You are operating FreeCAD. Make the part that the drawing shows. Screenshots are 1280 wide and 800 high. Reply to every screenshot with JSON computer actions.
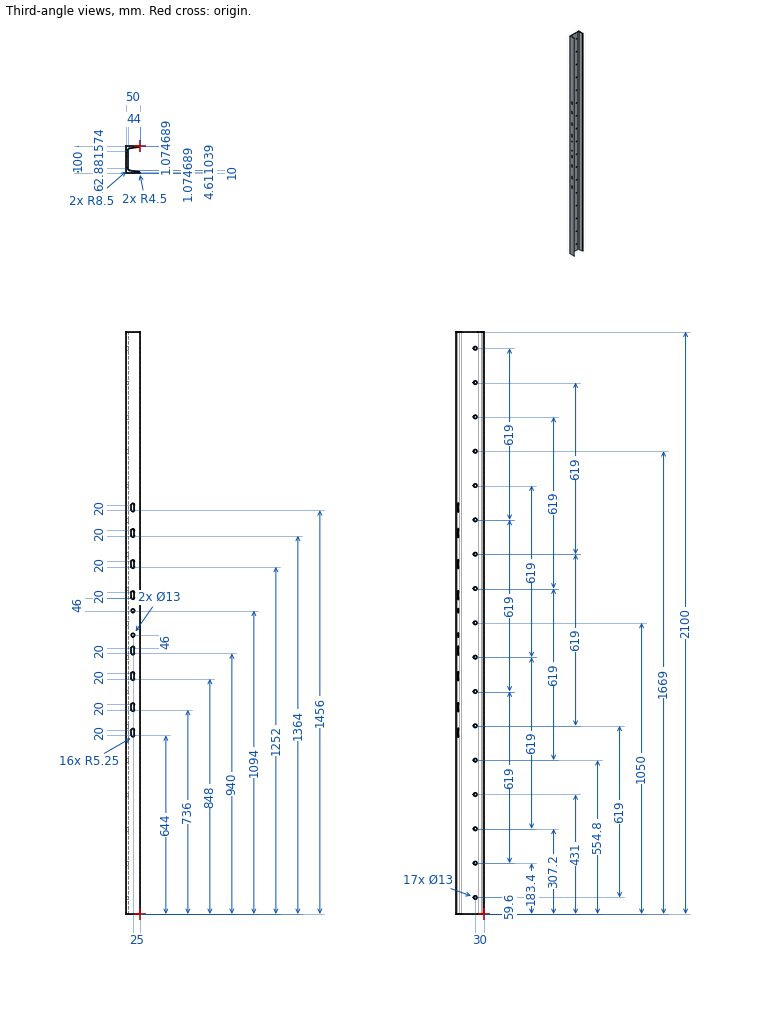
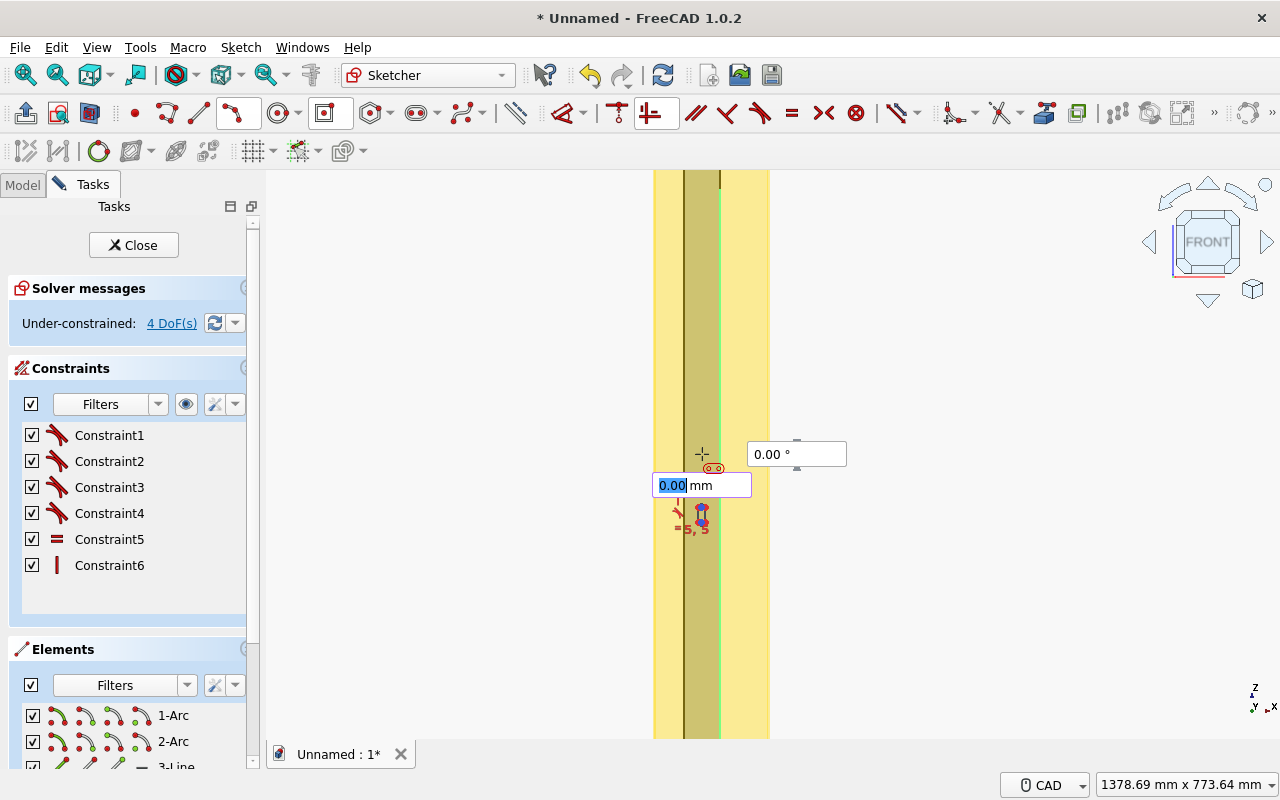
{"action": "left_click", "coordinate": [702, 439]}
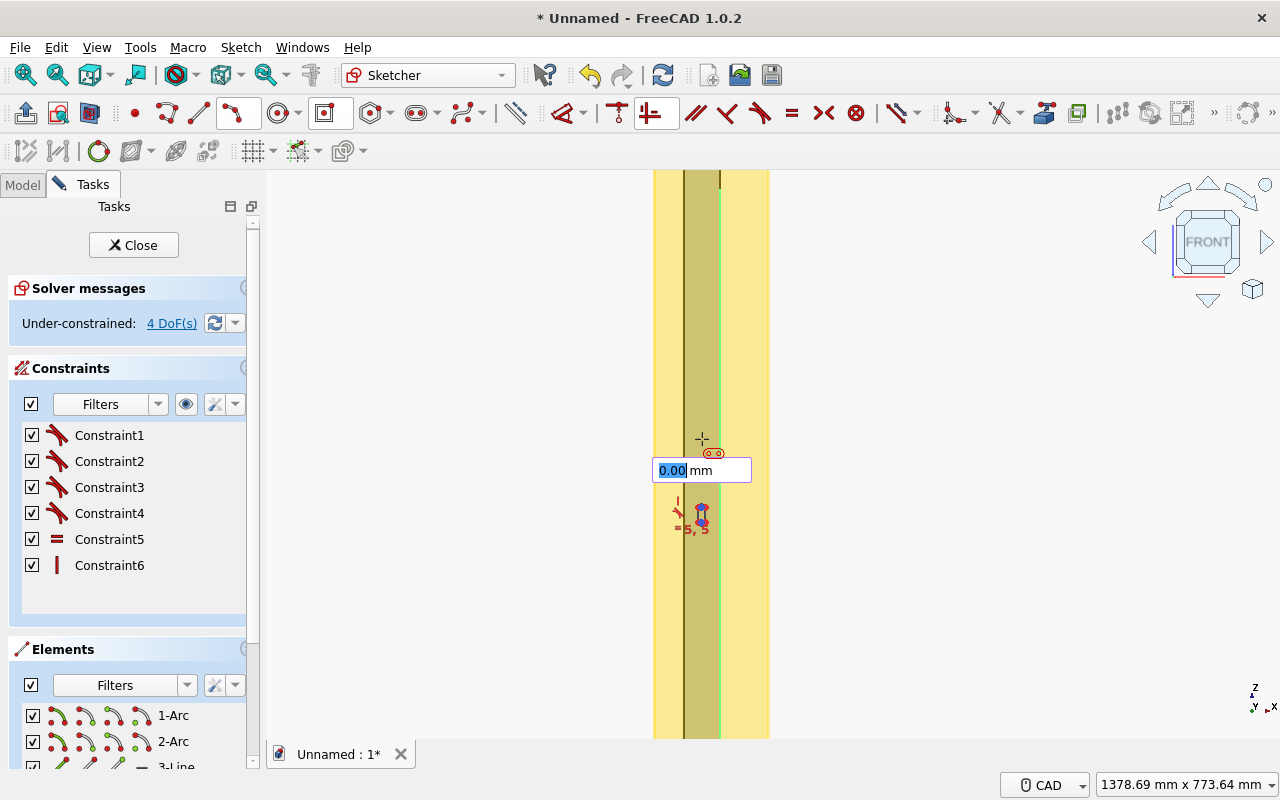
{"action": "scroll", "coordinate": [698, 447], "scroll_direction": "up", "scroll_amount": 8}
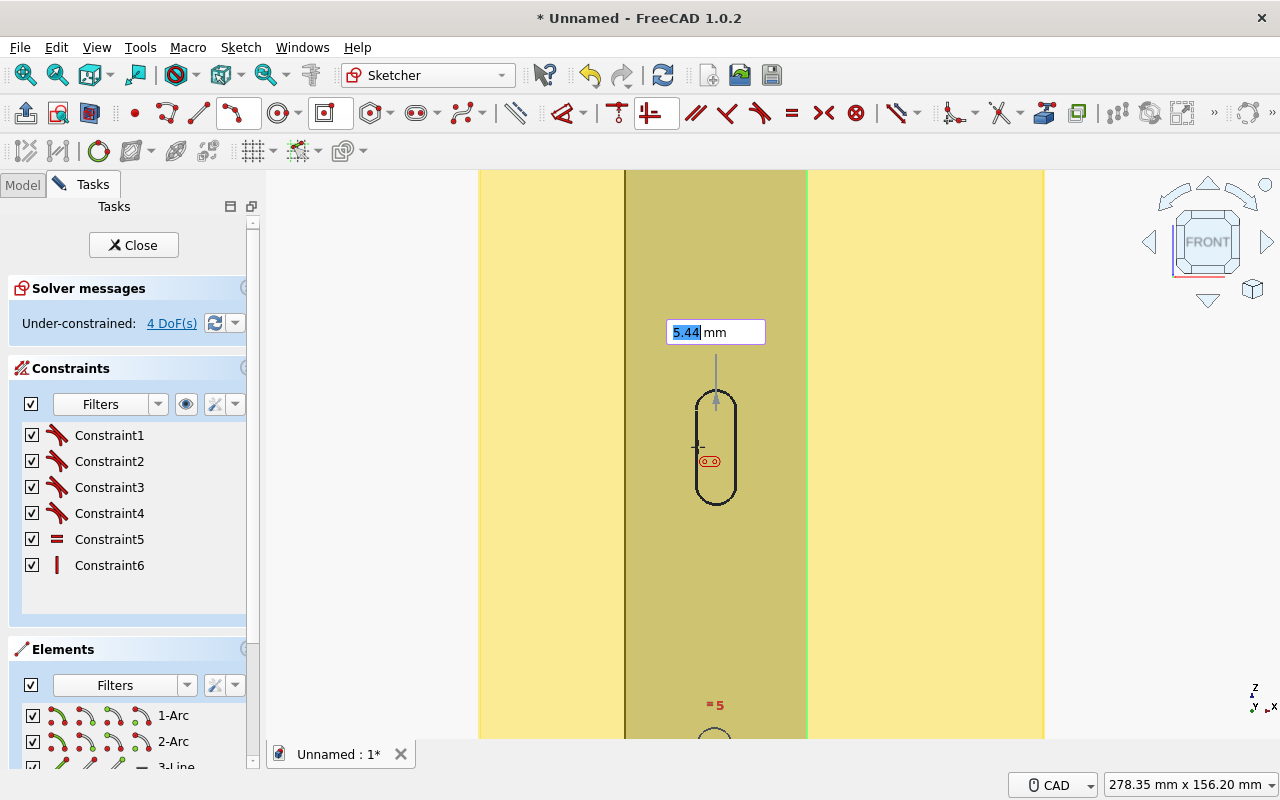
{"action": "left_click", "coordinate": [697, 443]}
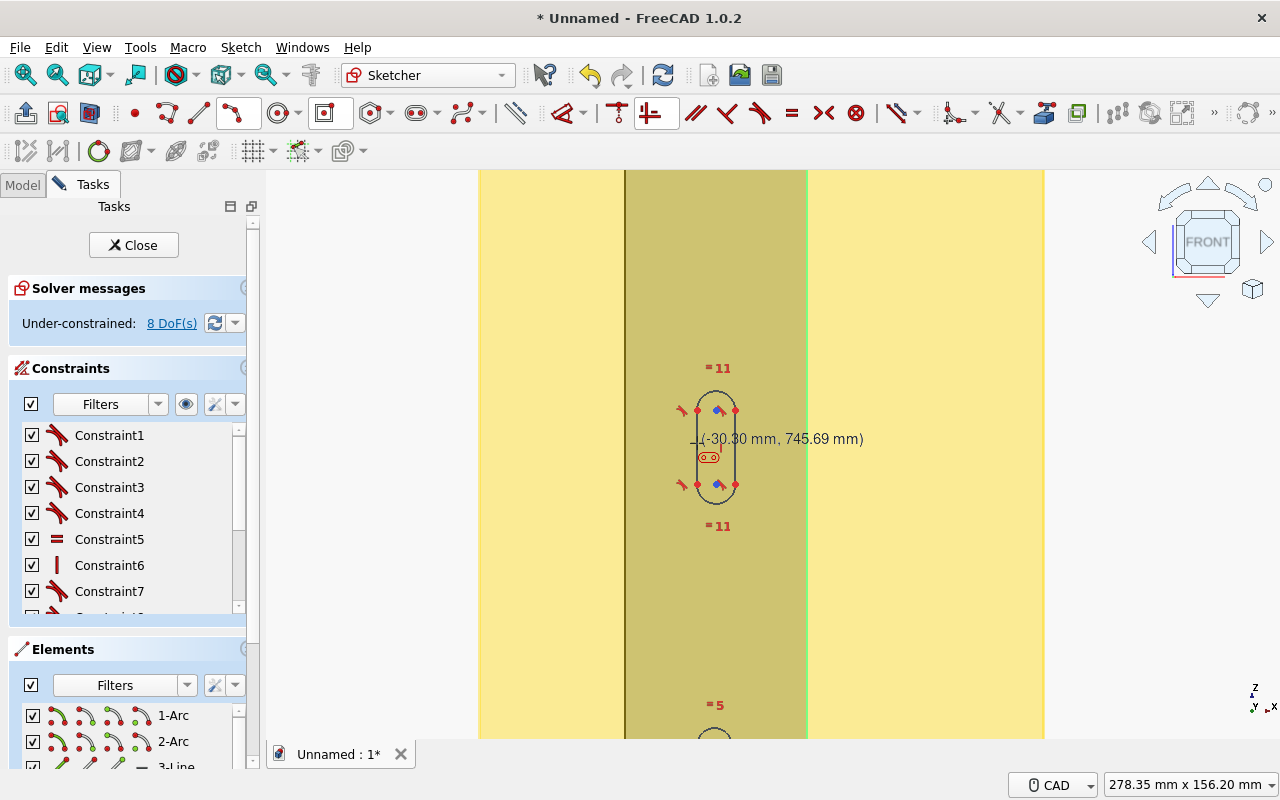
{"action": "scroll", "coordinate": [702, 454], "scroll_direction": "down", "scroll_amount": 14}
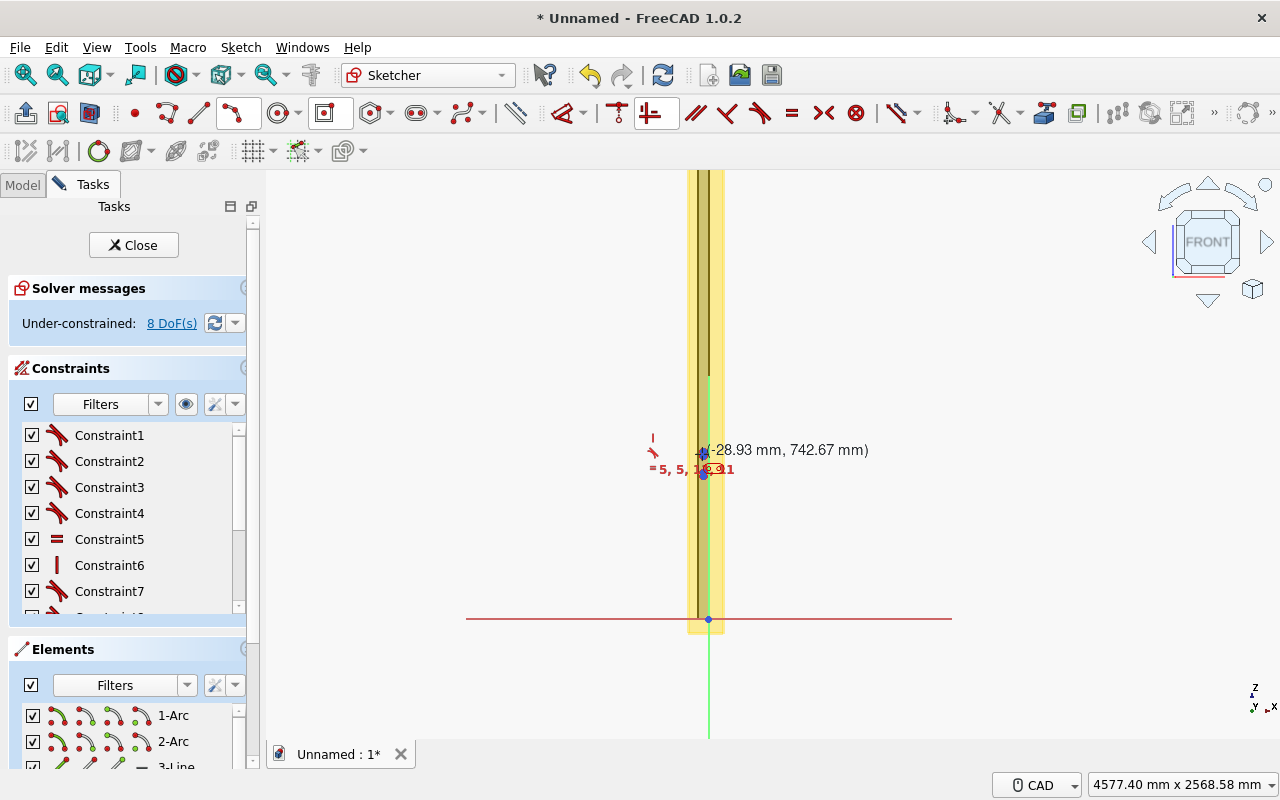
{"action": "scroll", "coordinate": [703, 431], "scroll_direction": "up", "scroll_amount": 15}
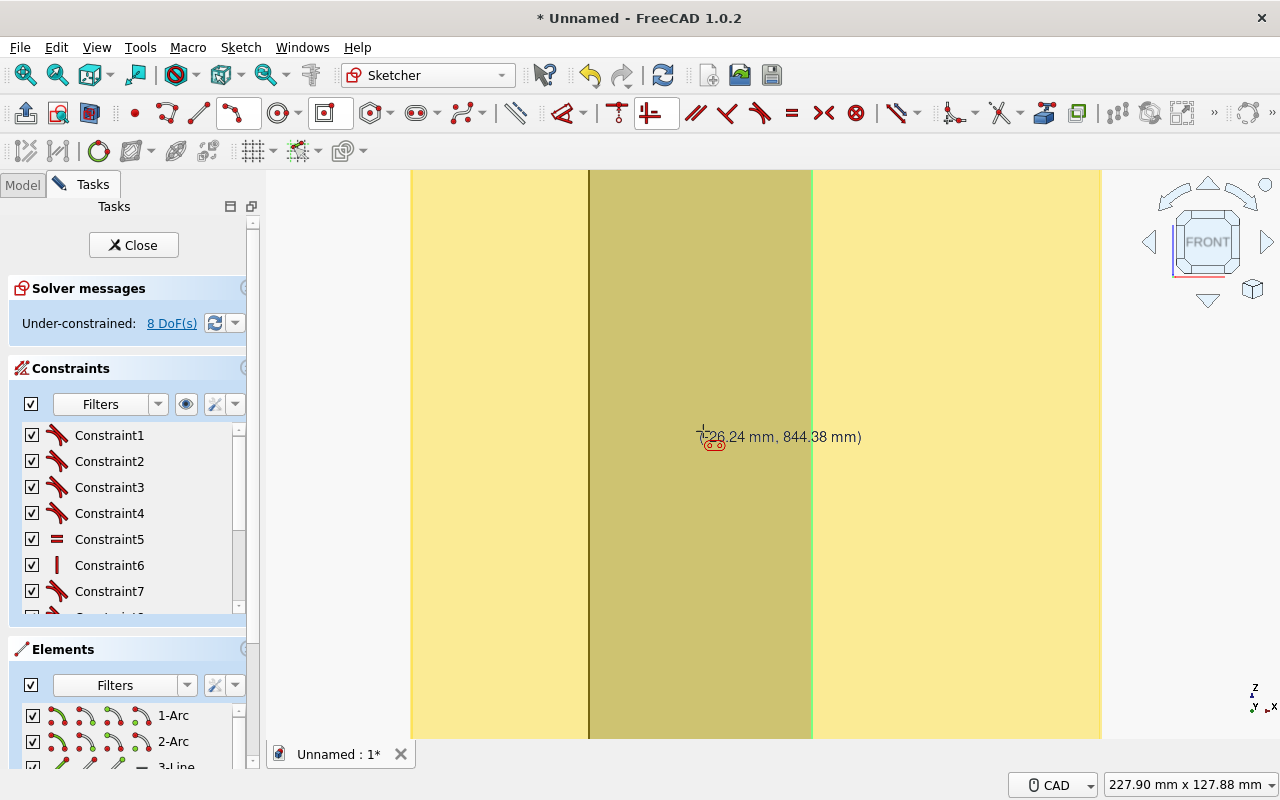
{"action": "scroll", "coordinate": [703, 431], "scroll_direction": "down", "scroll_amount": 15}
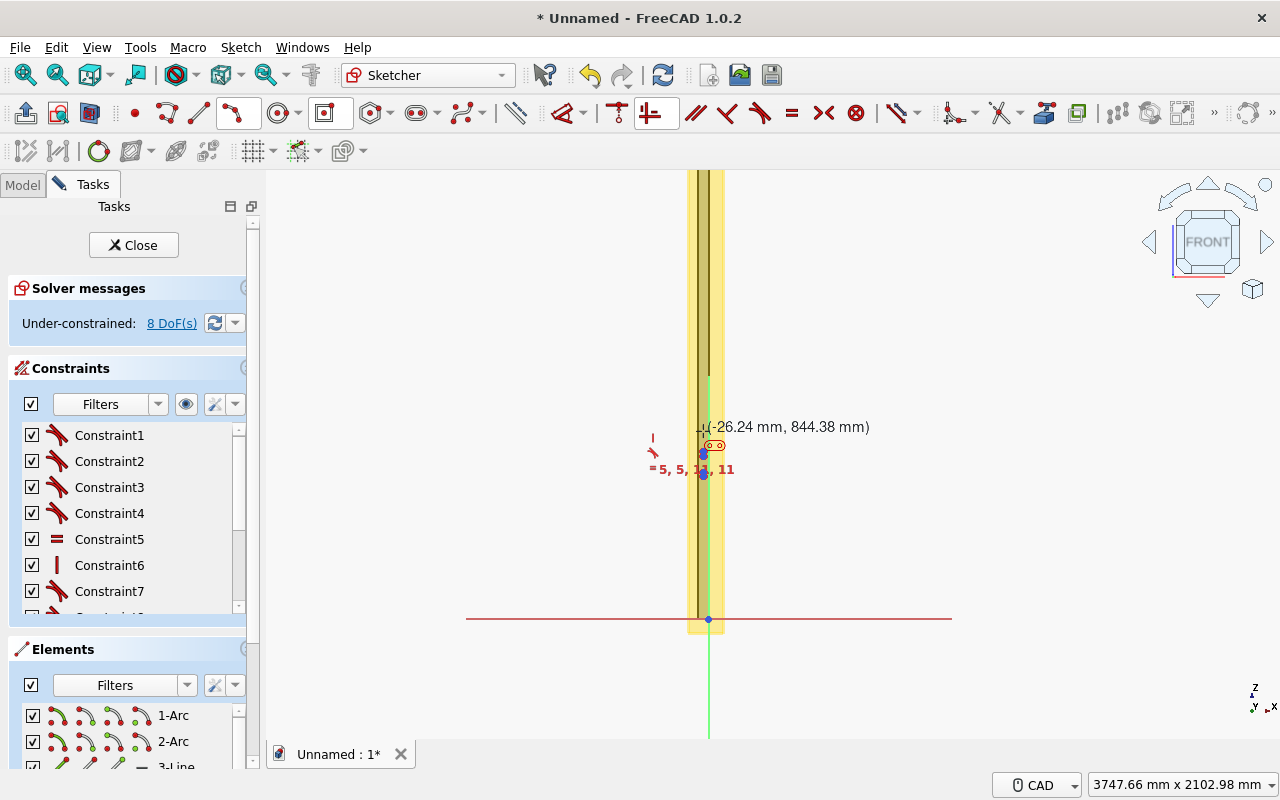
{"action": "scroll", "coordinate": [703, 431], "scroll_direction": "up", "scroll_amount": 6}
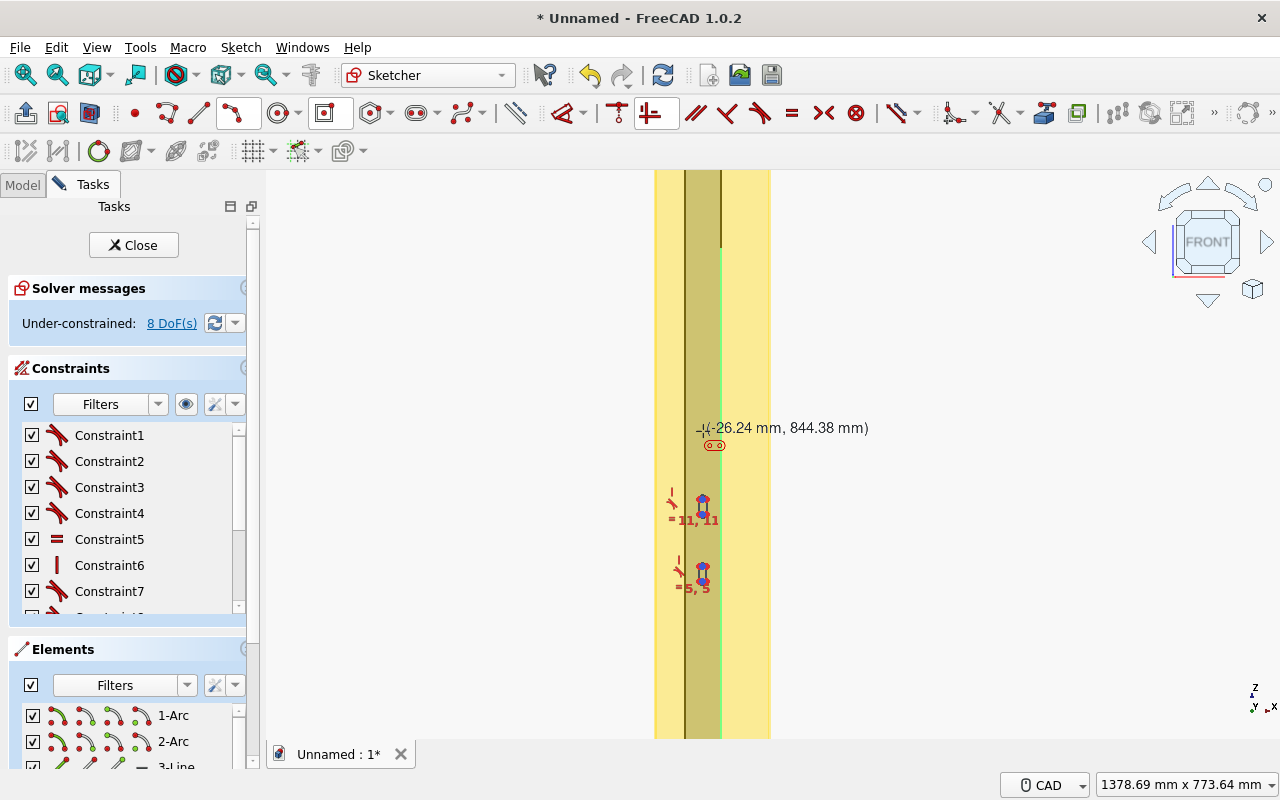
{"action": "left_click", "coordinate": [703, 431]}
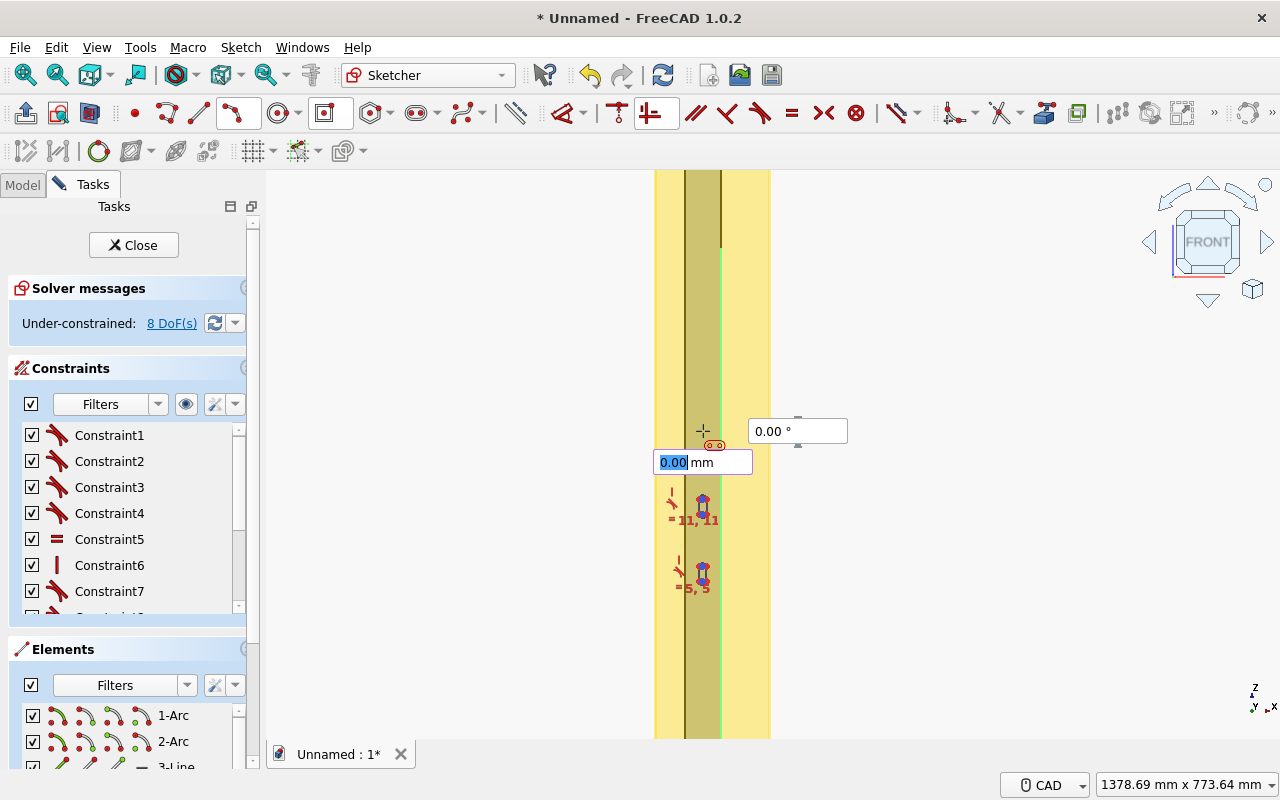
{"action": "left_click", "coordinate": [703, 416]}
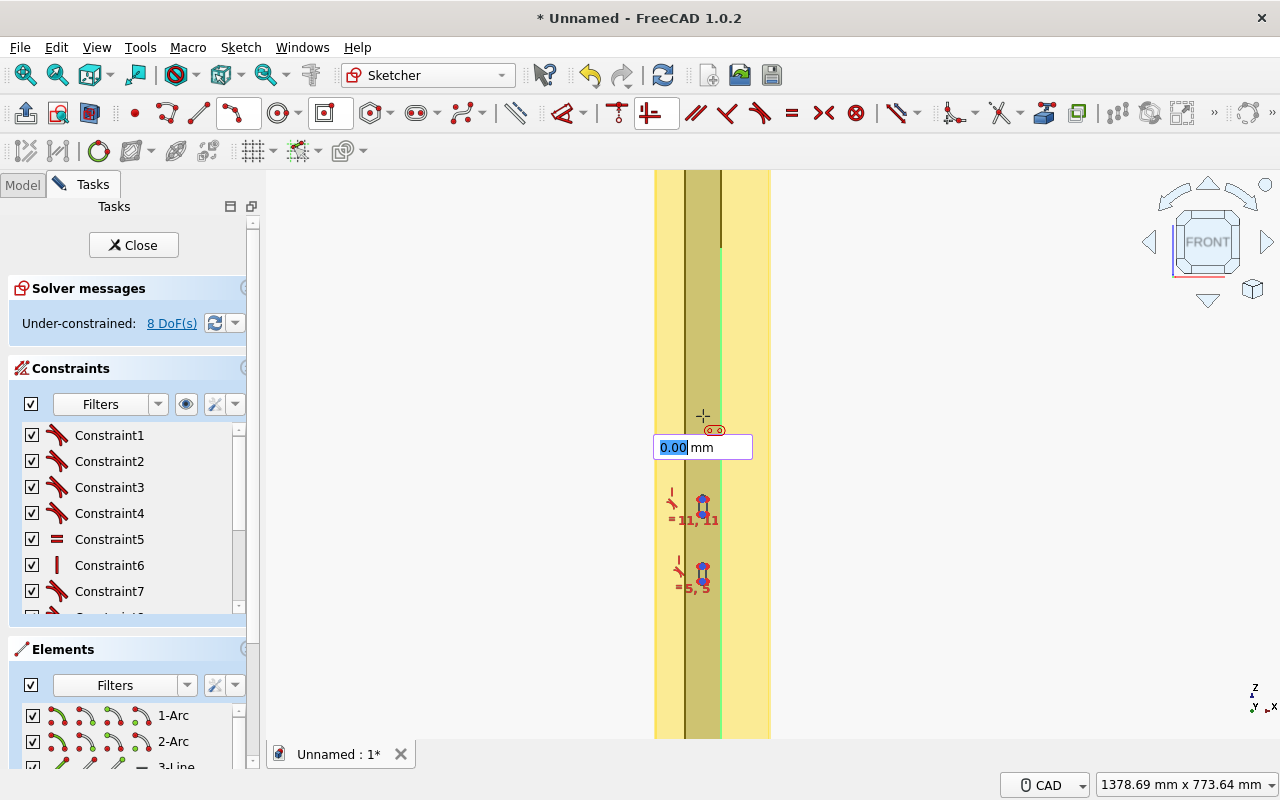
{"action": "scroll", "coordinate": [707, 423], "scroll_direction": "up", "scroll_amount": 8}